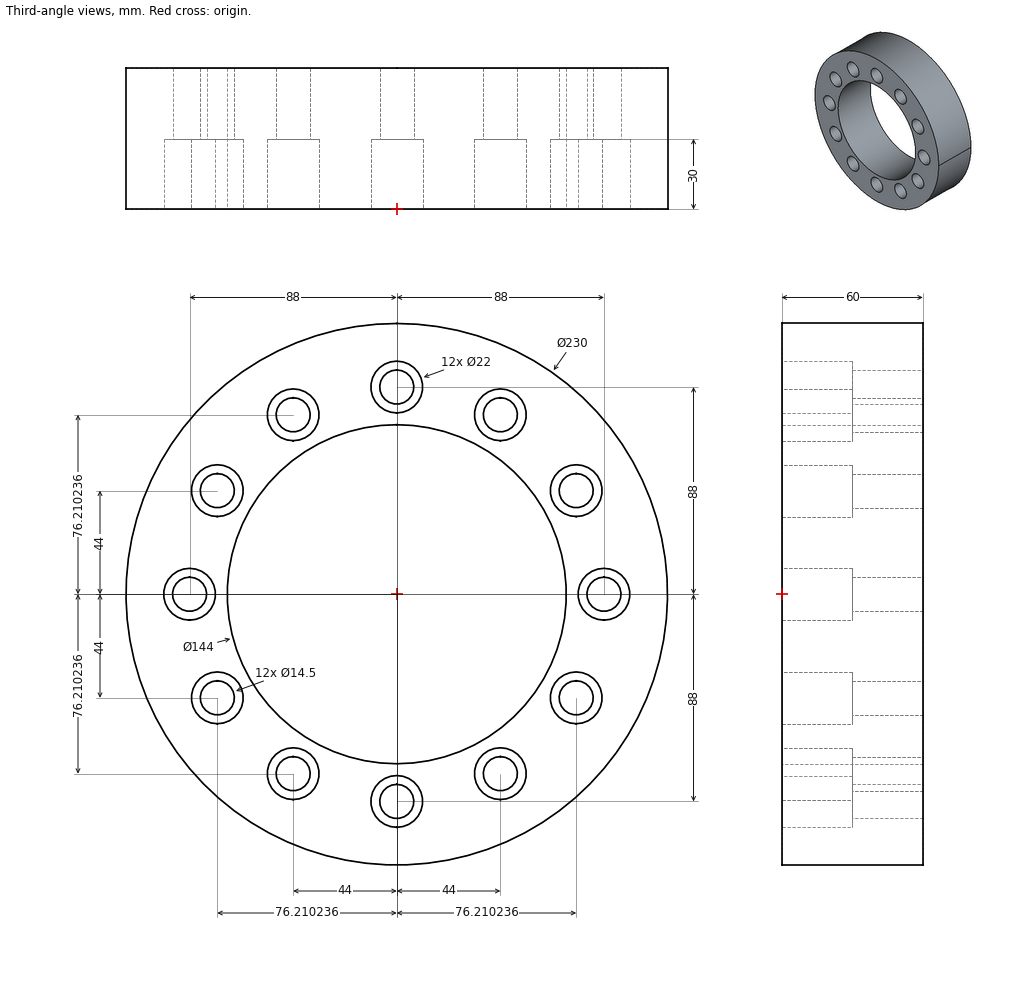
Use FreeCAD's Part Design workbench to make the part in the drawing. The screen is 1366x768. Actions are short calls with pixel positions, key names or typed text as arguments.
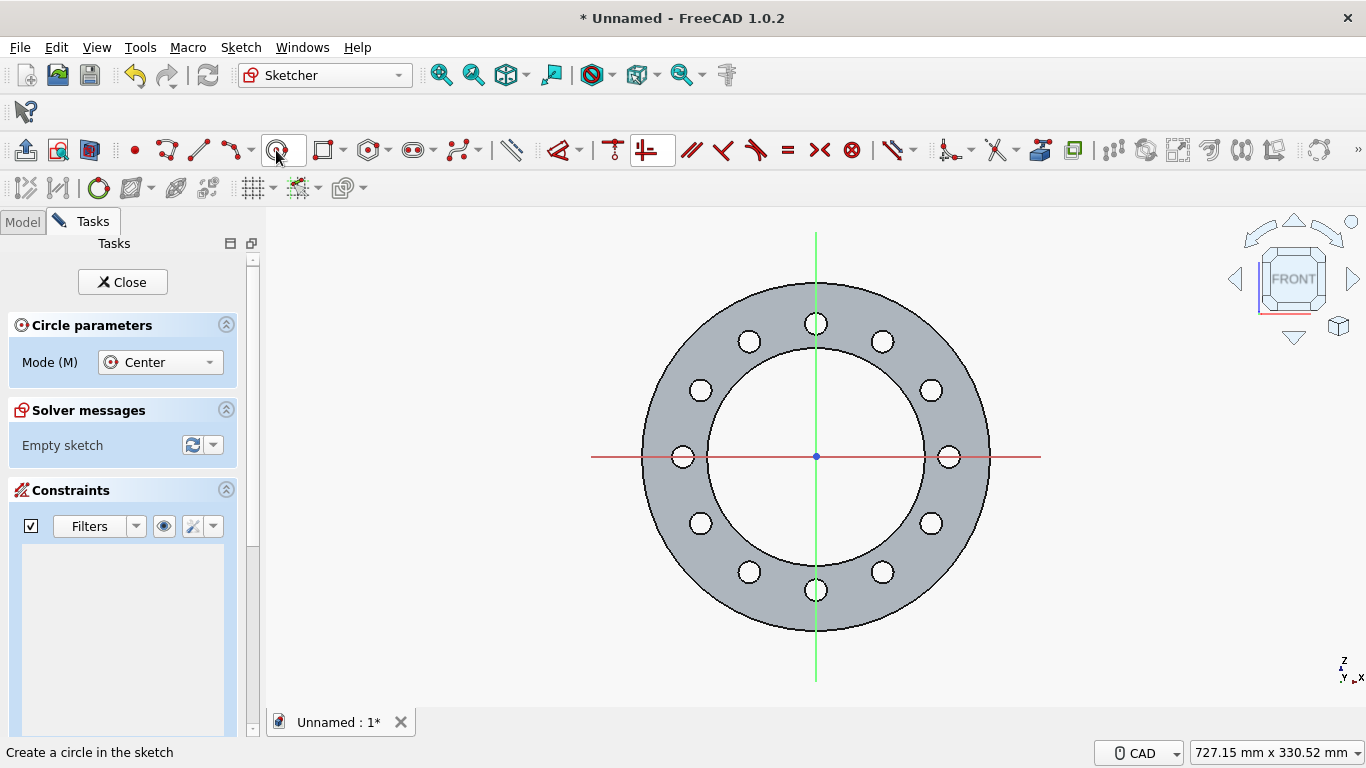
scroll(816, 324, up, 2)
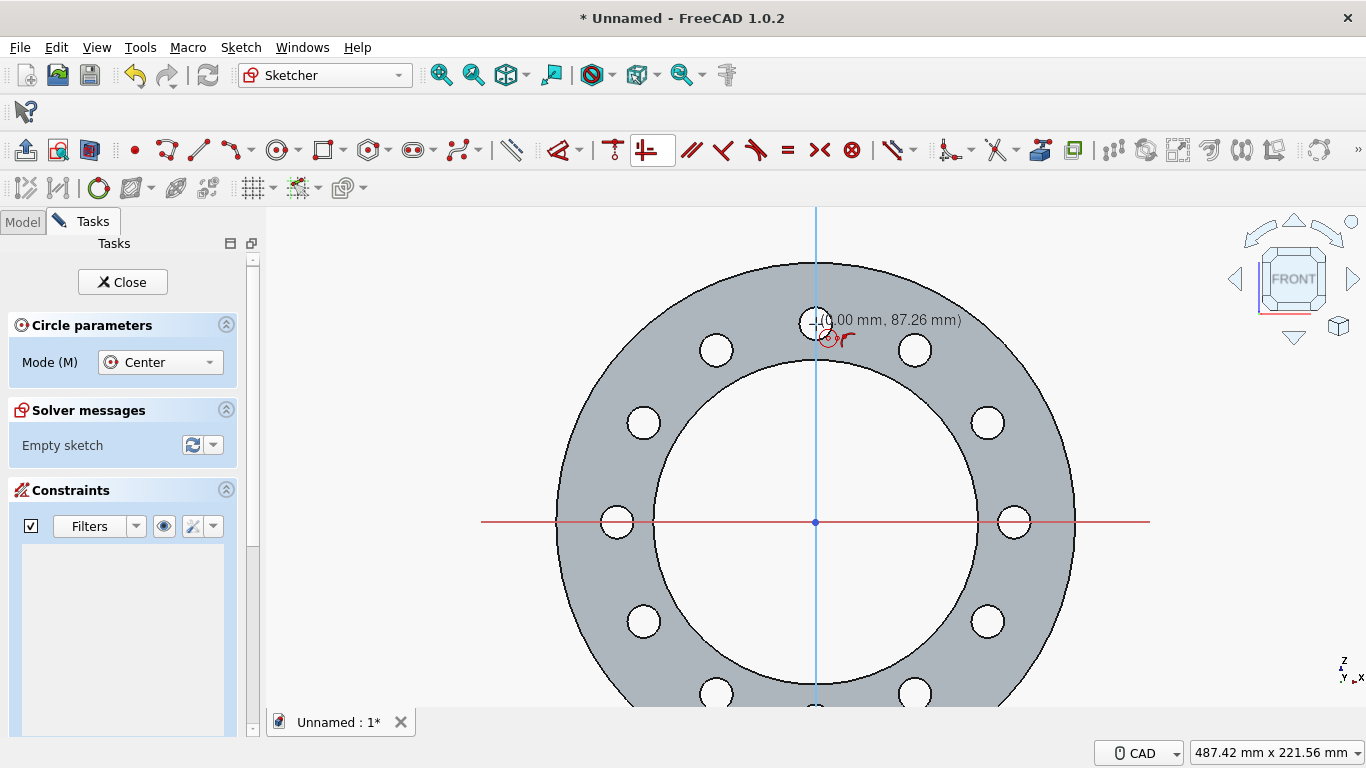
click(816, 324)
move(833, 306)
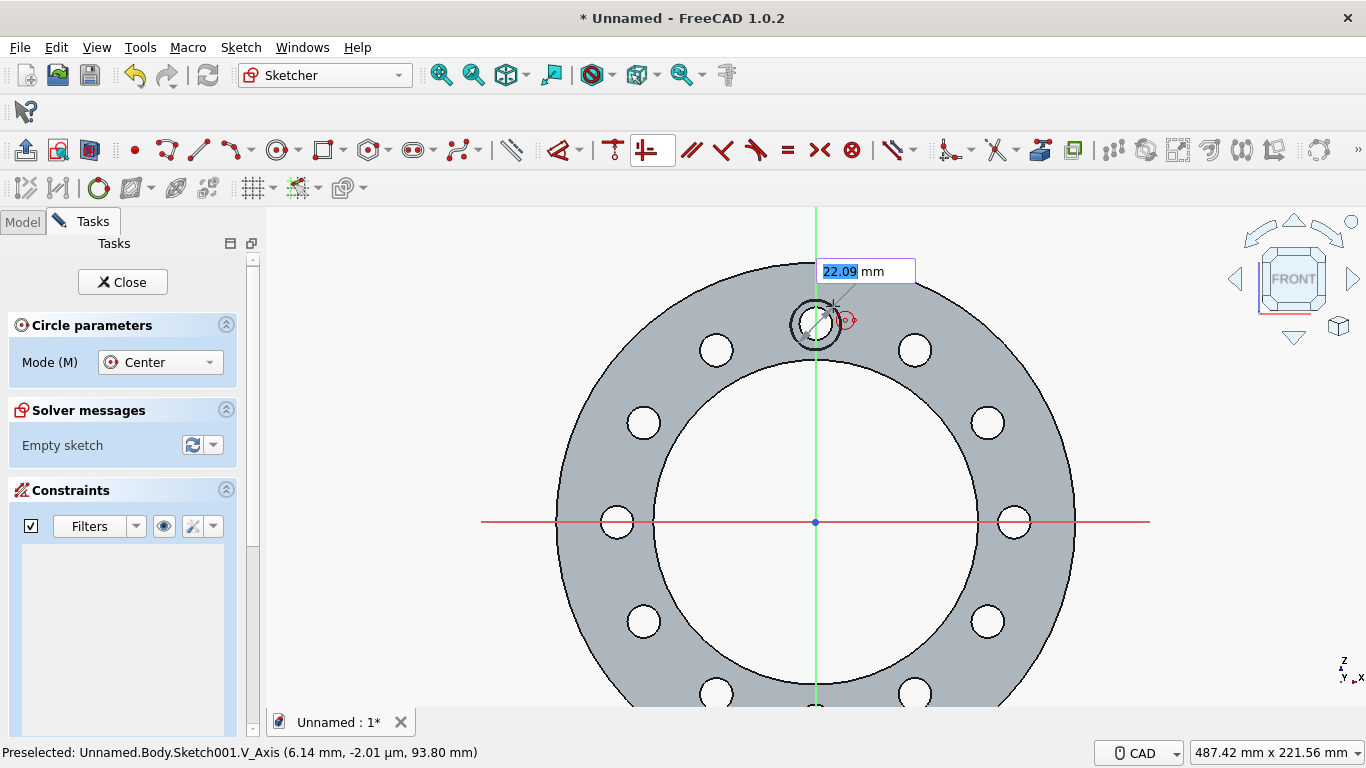
text(22)
key(Return)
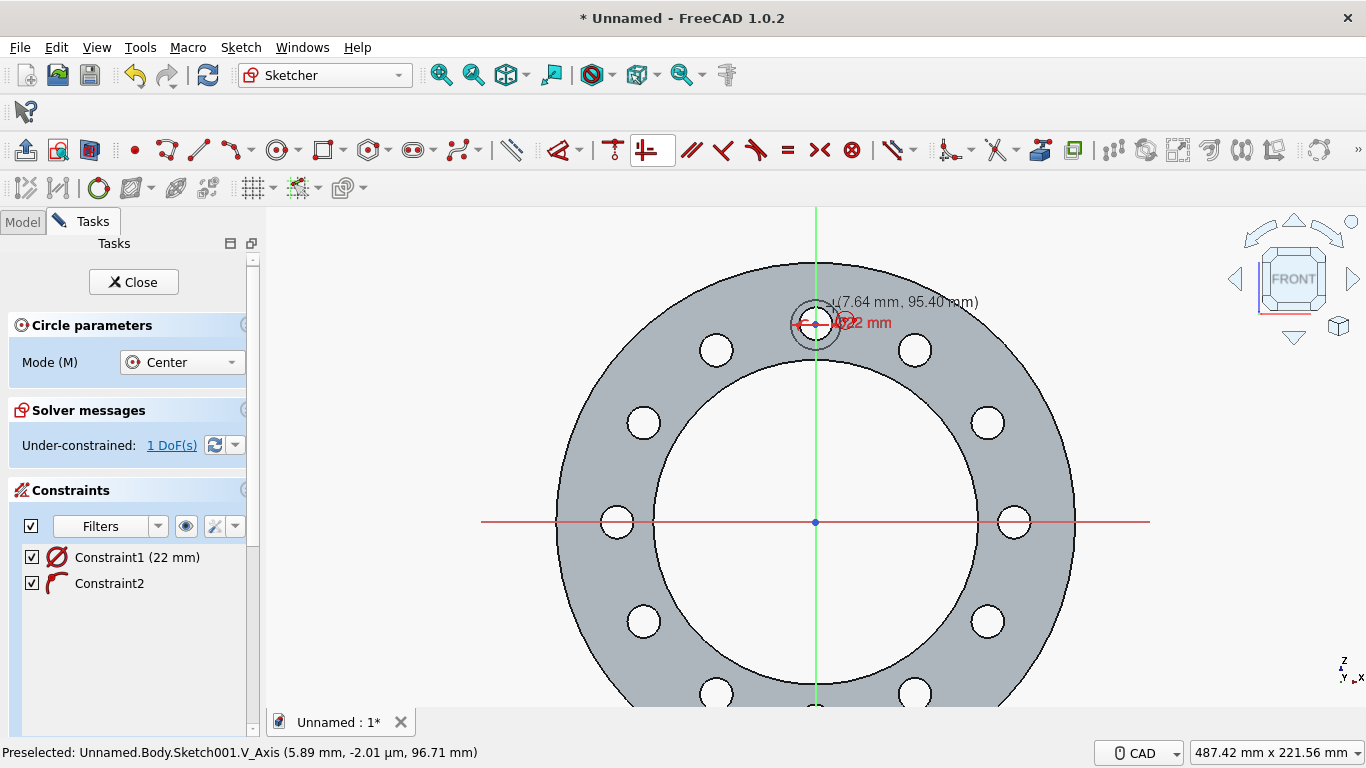
click(915, 350)
move(933, 333)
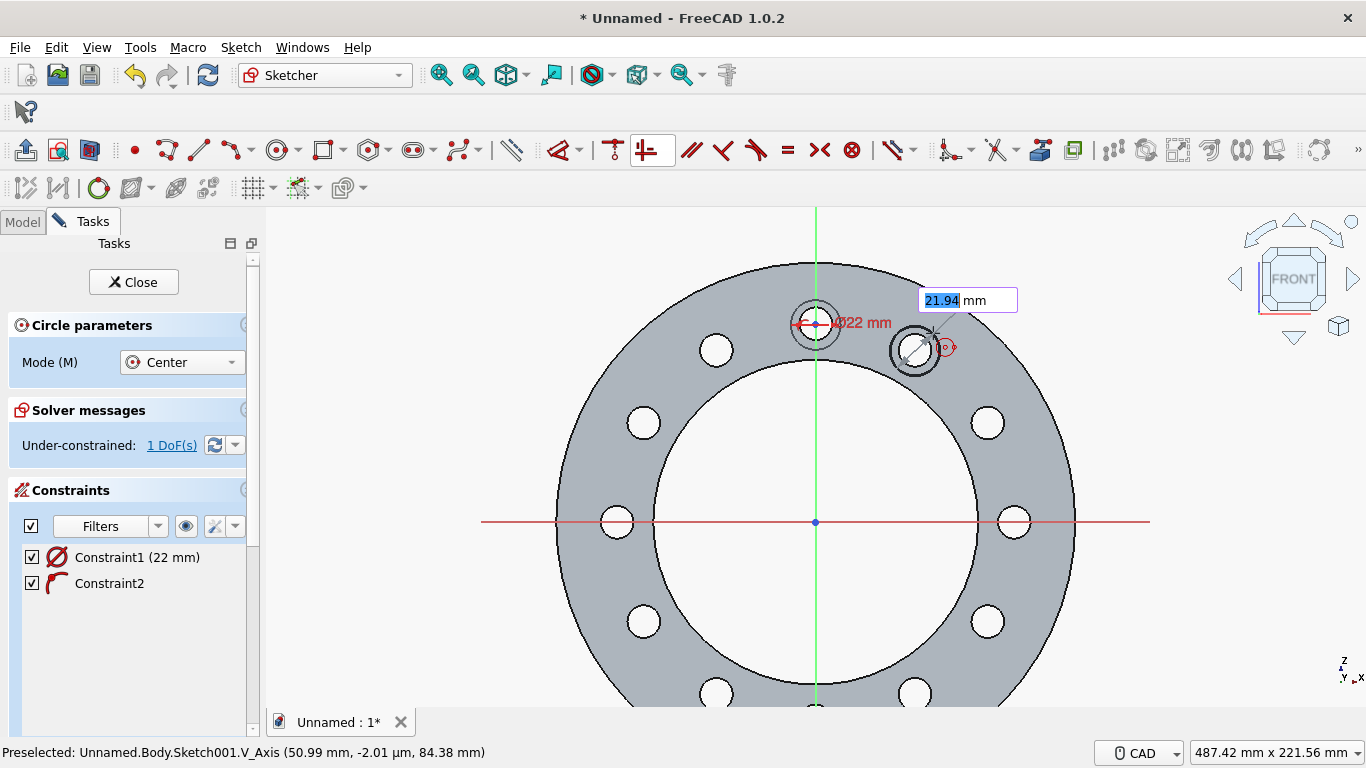
text(22)
key(Return)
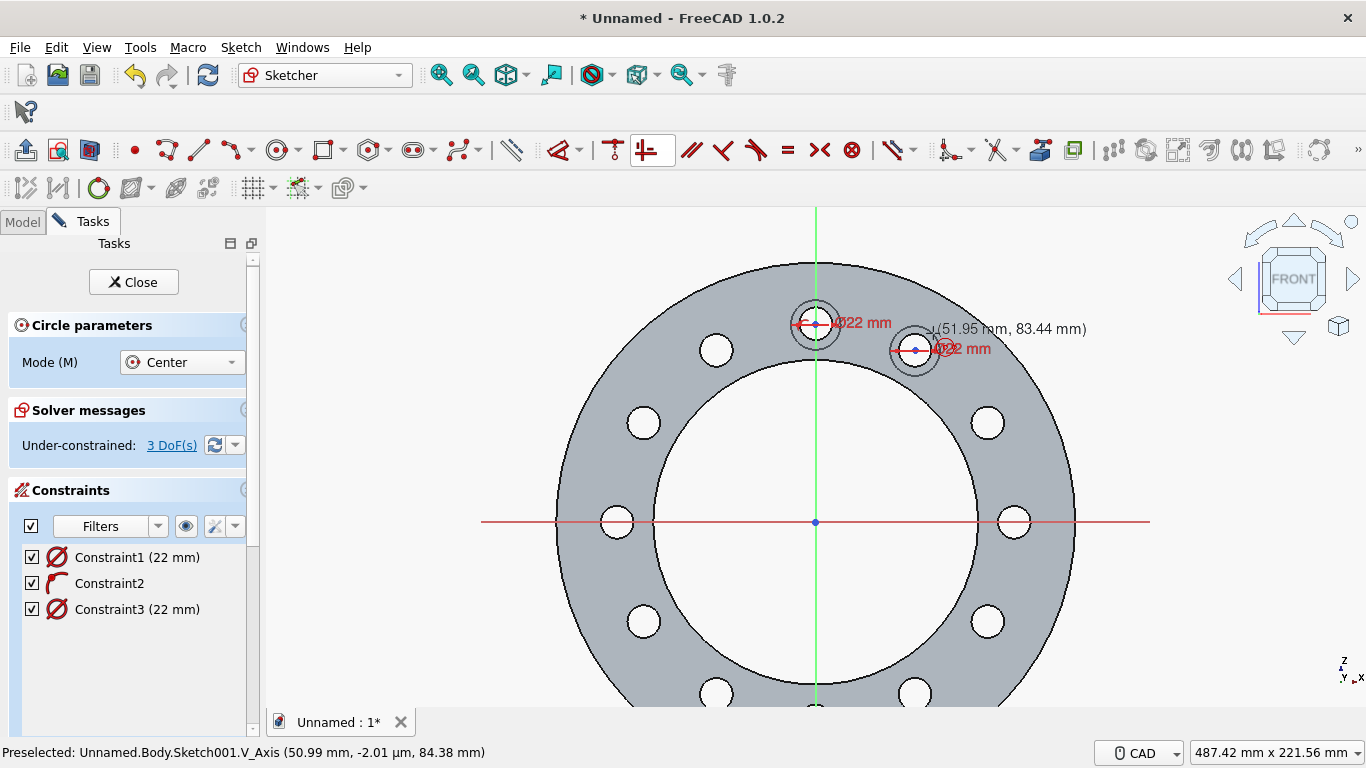
click(988, 423)
move(1005, 405)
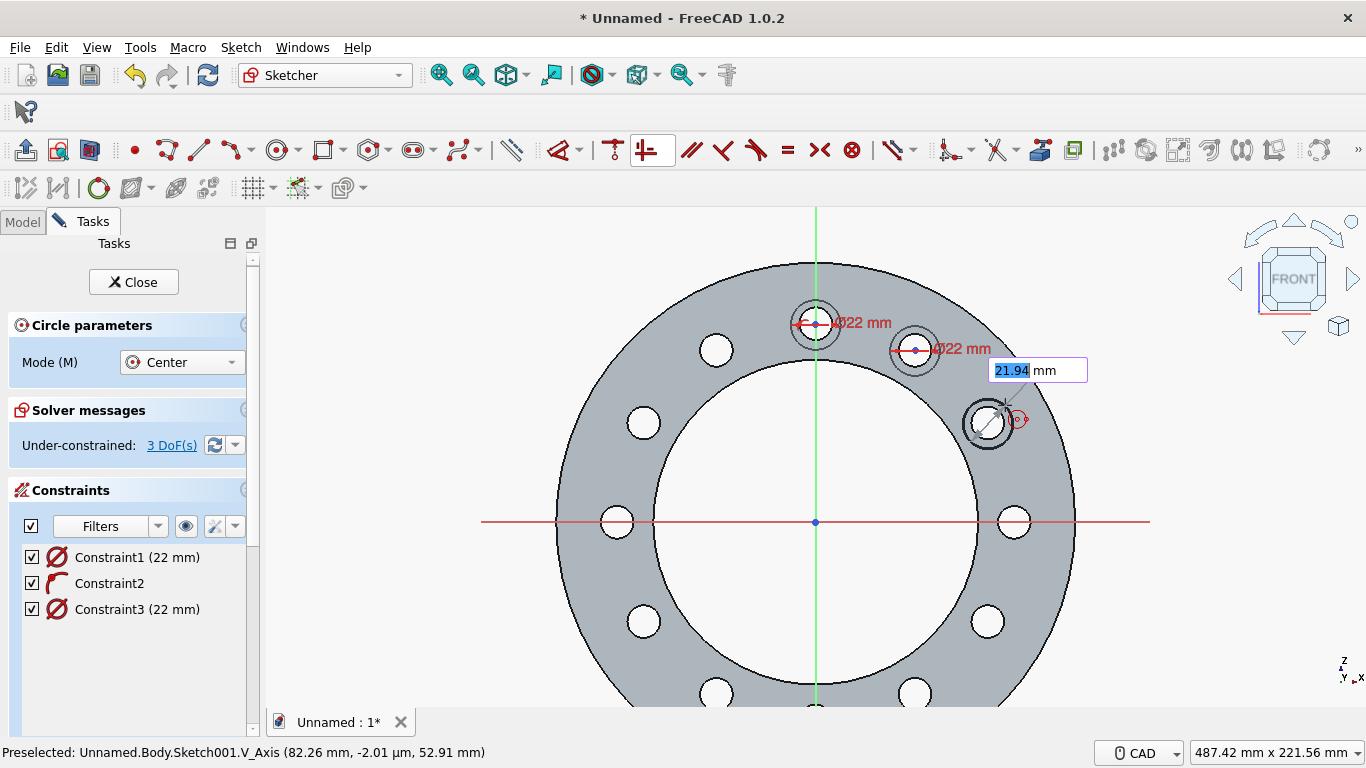
text(22)
key(Return)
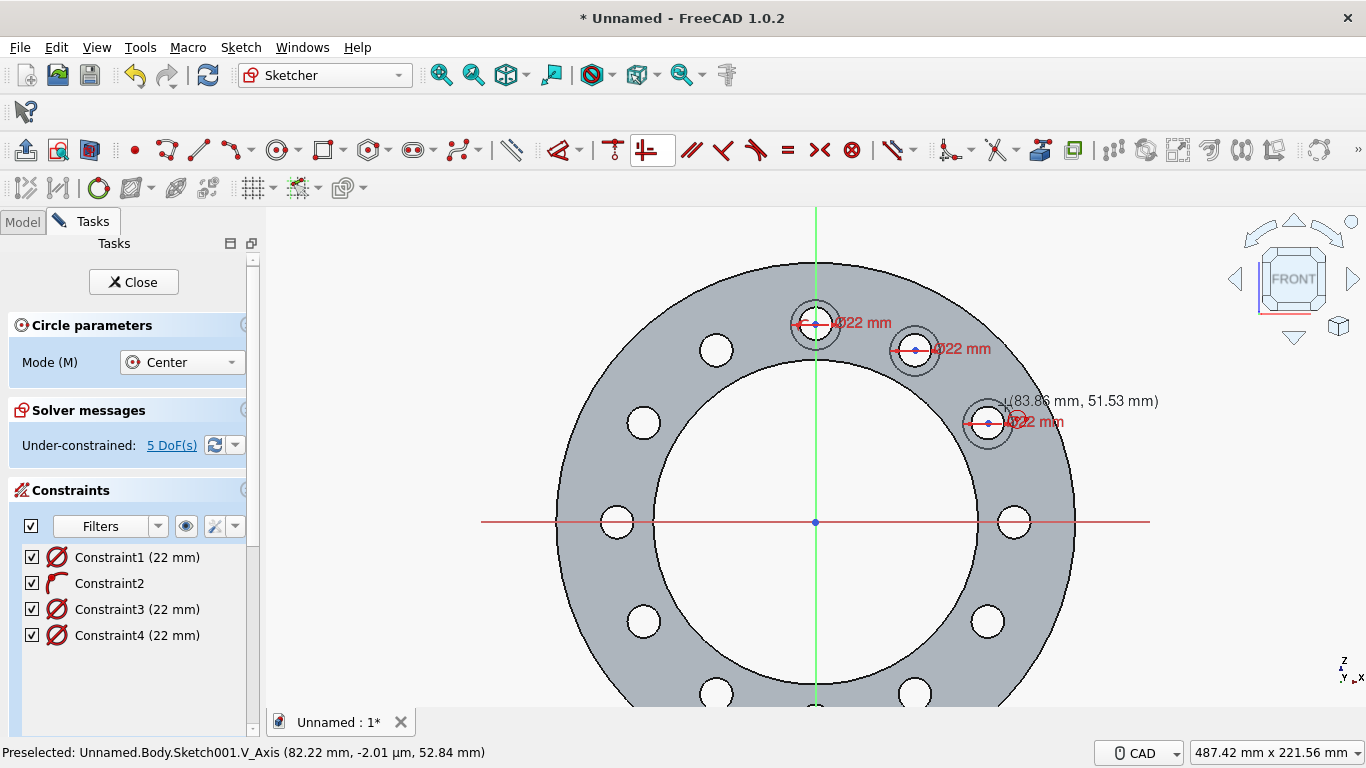
click(1014, 522)
move(1032, 505)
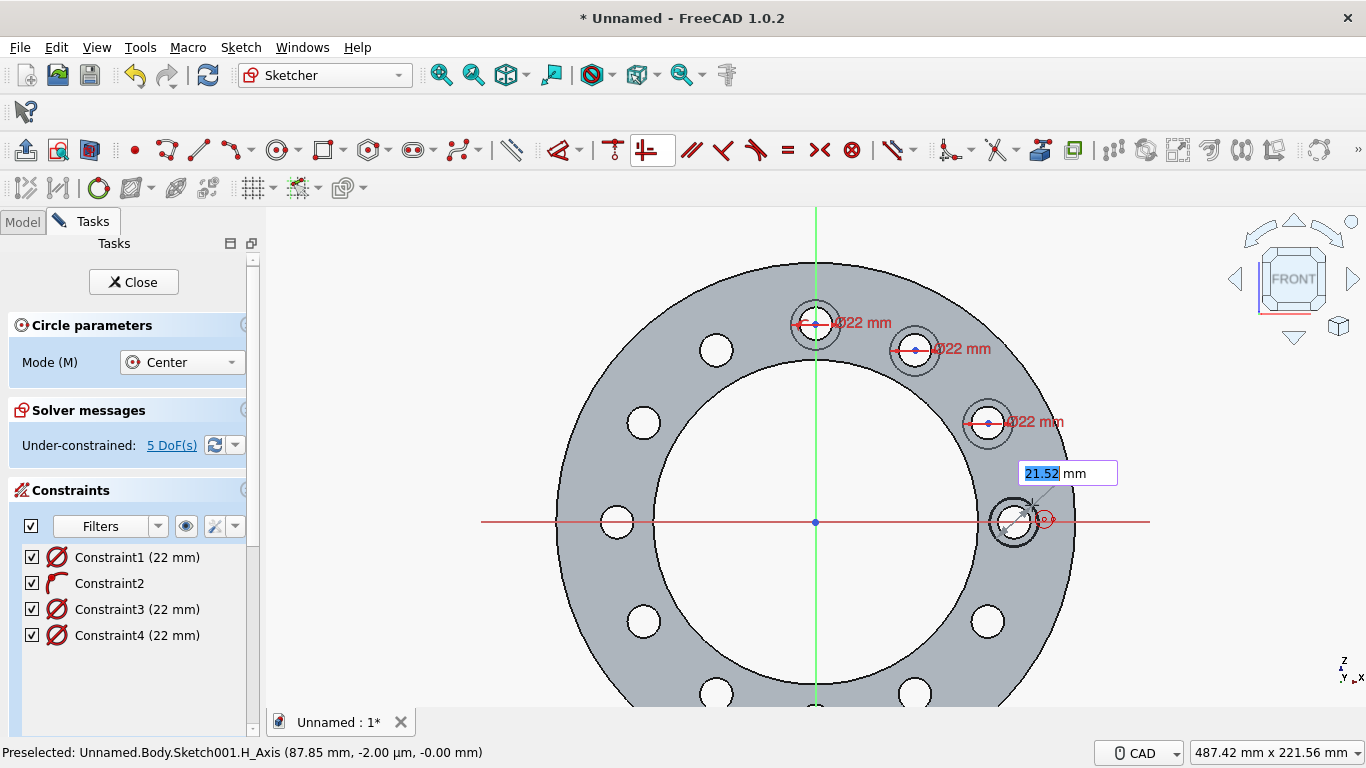
text(22)
key(Return)